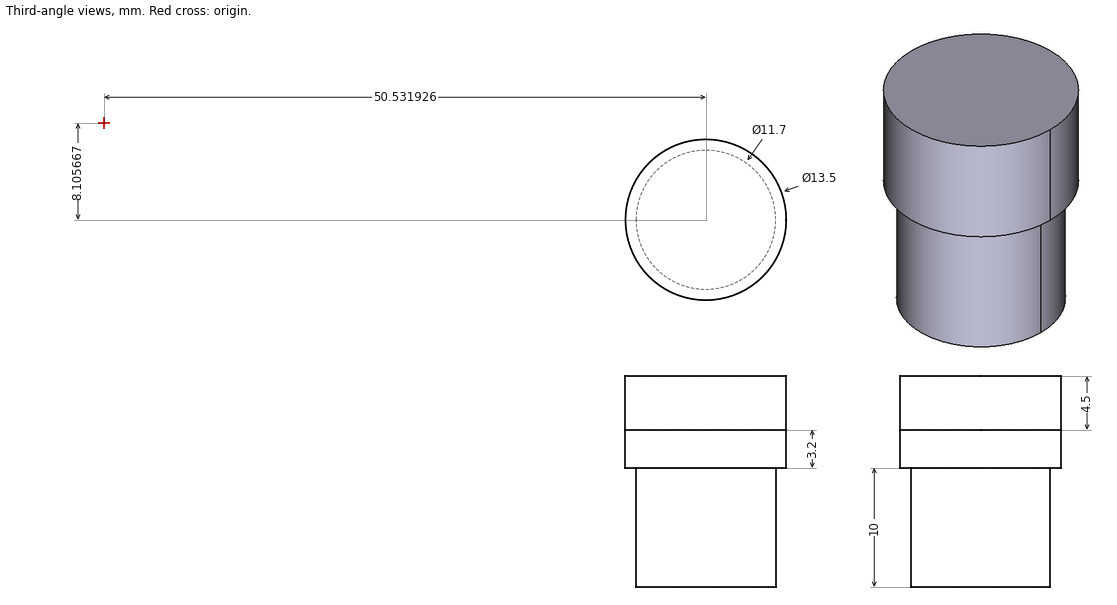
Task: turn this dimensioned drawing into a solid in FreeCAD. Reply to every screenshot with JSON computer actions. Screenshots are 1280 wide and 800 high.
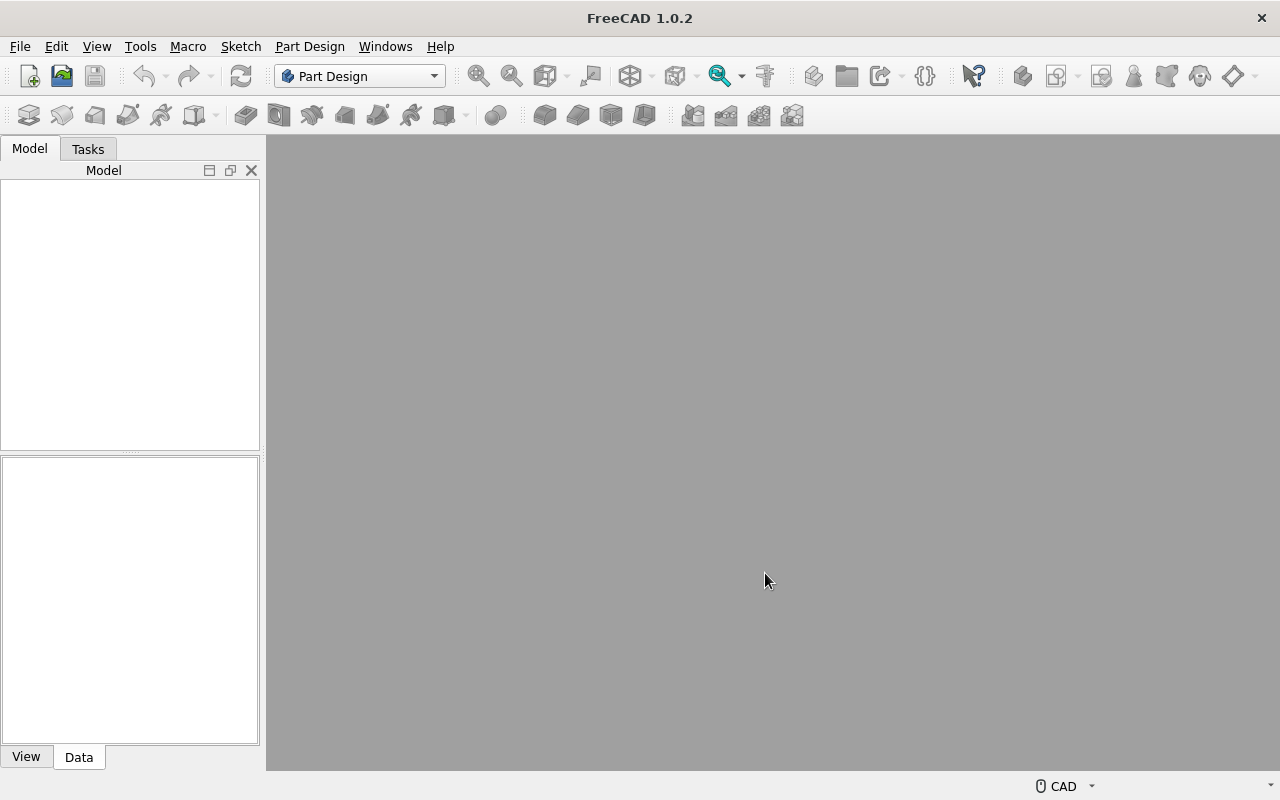
{"action": "key", "text": "ctrl+n"}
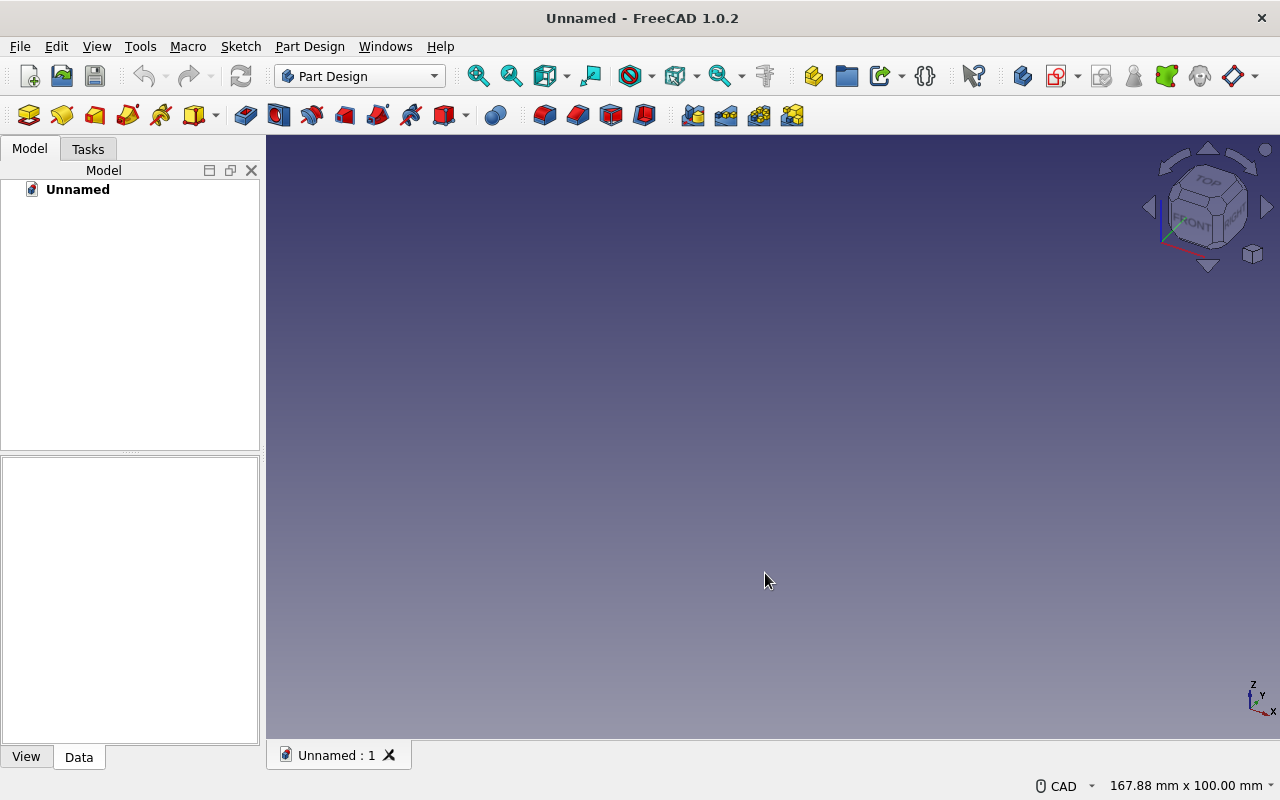
{"action": "left_click", "coordinate": [1056, 76]}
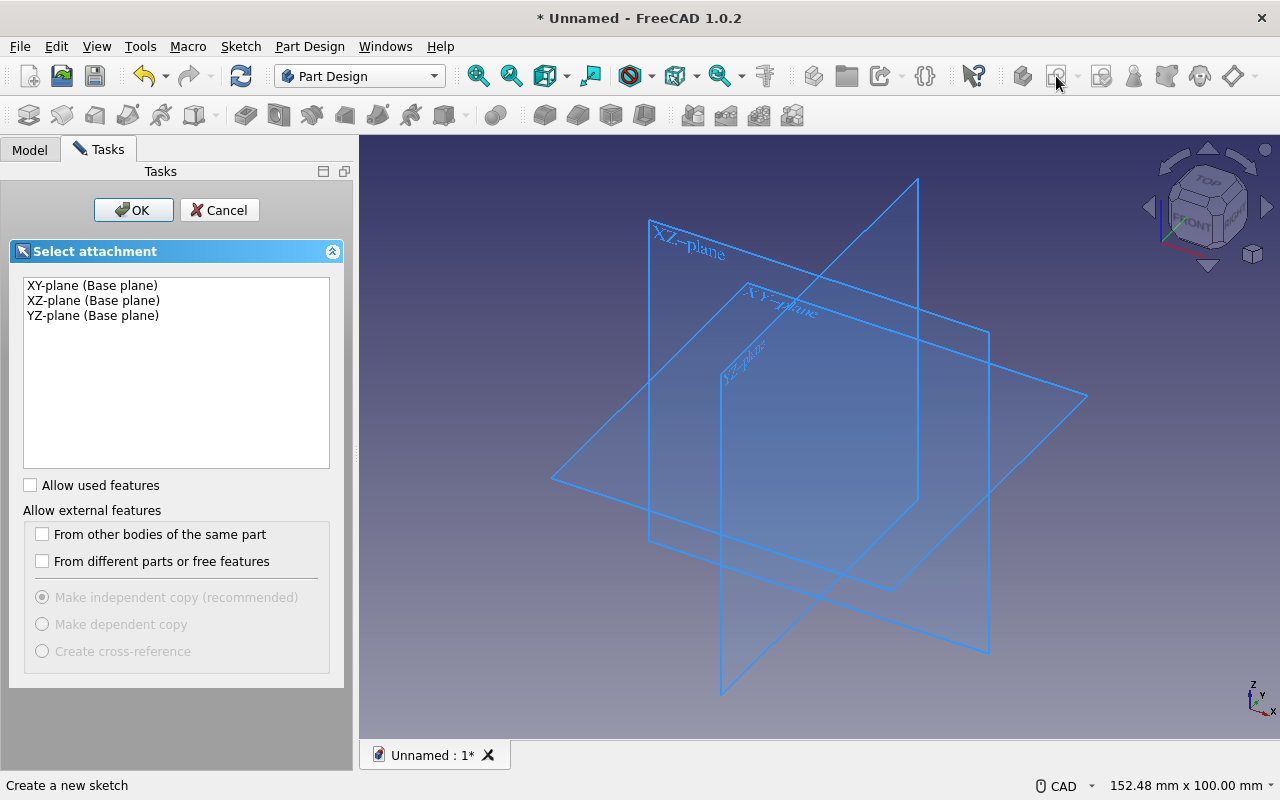
{"action": "left_click", "coordinate": [84, 286]}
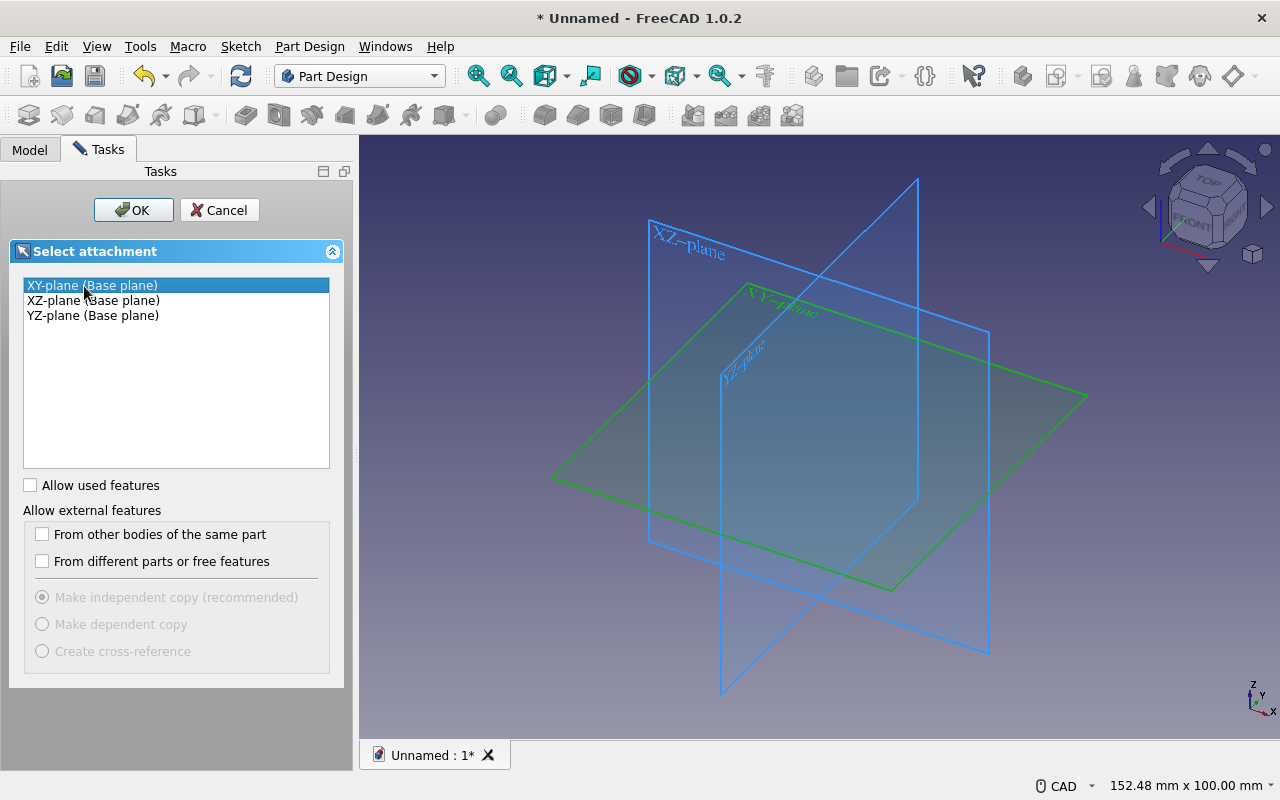
{"action": "left_click", "coordinate": [134, 210]}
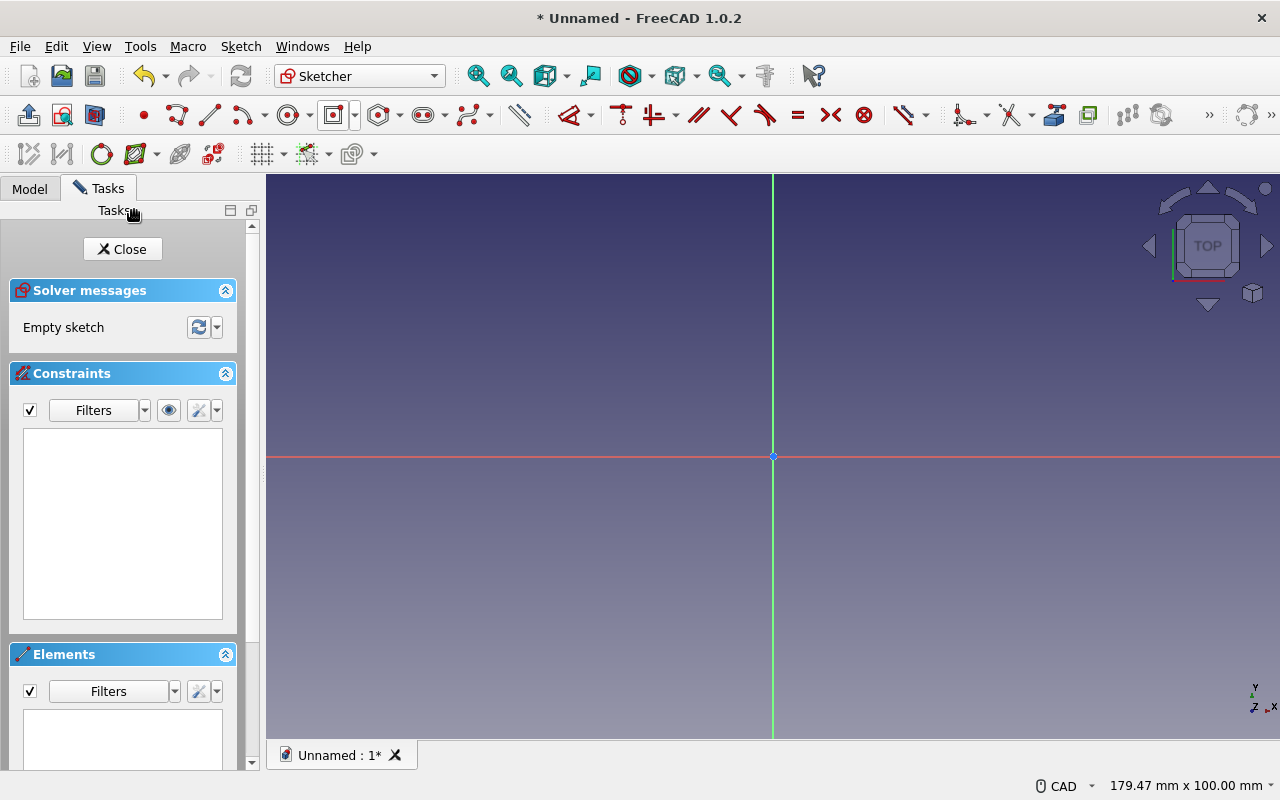
{"action": "scroll", "coordinate": [1115, 514], "scroll_direction": "up", "scroll_amount": 8}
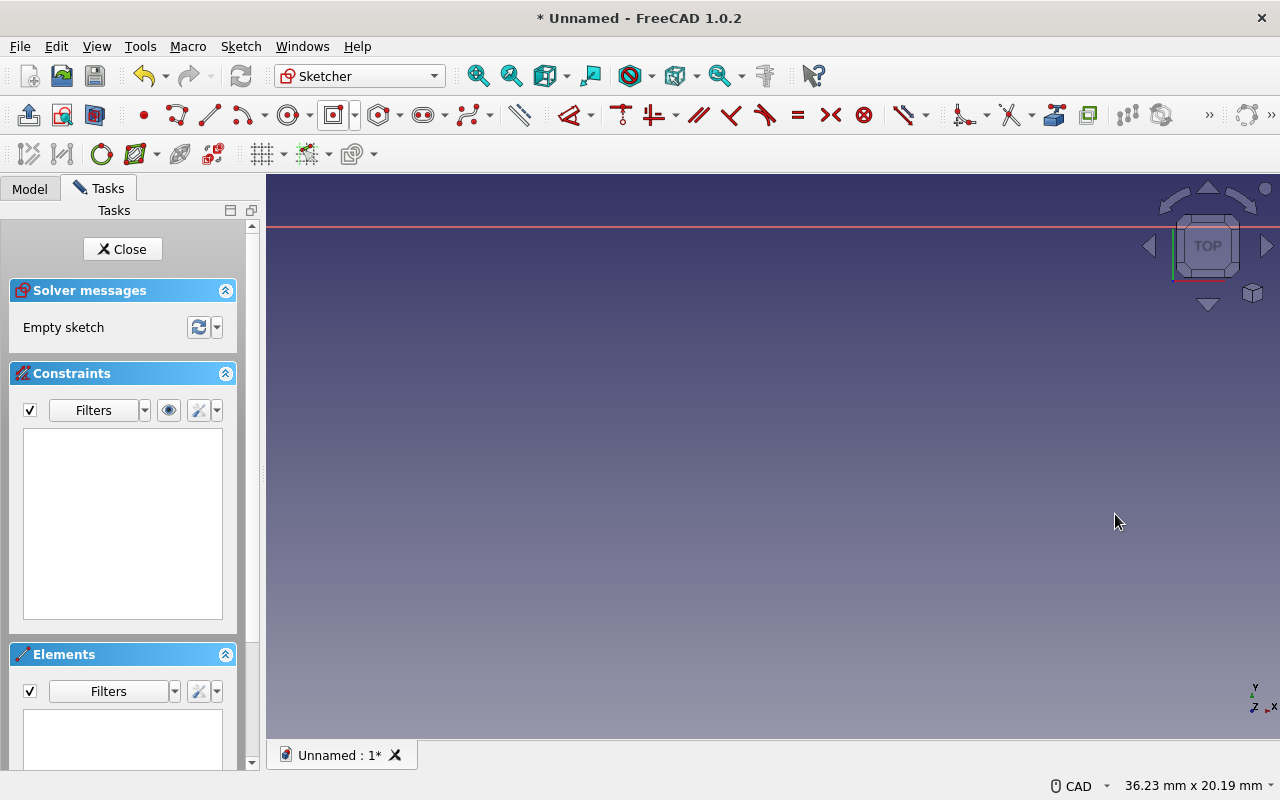
{"action": "left_click", "coordinate": [288, 116]}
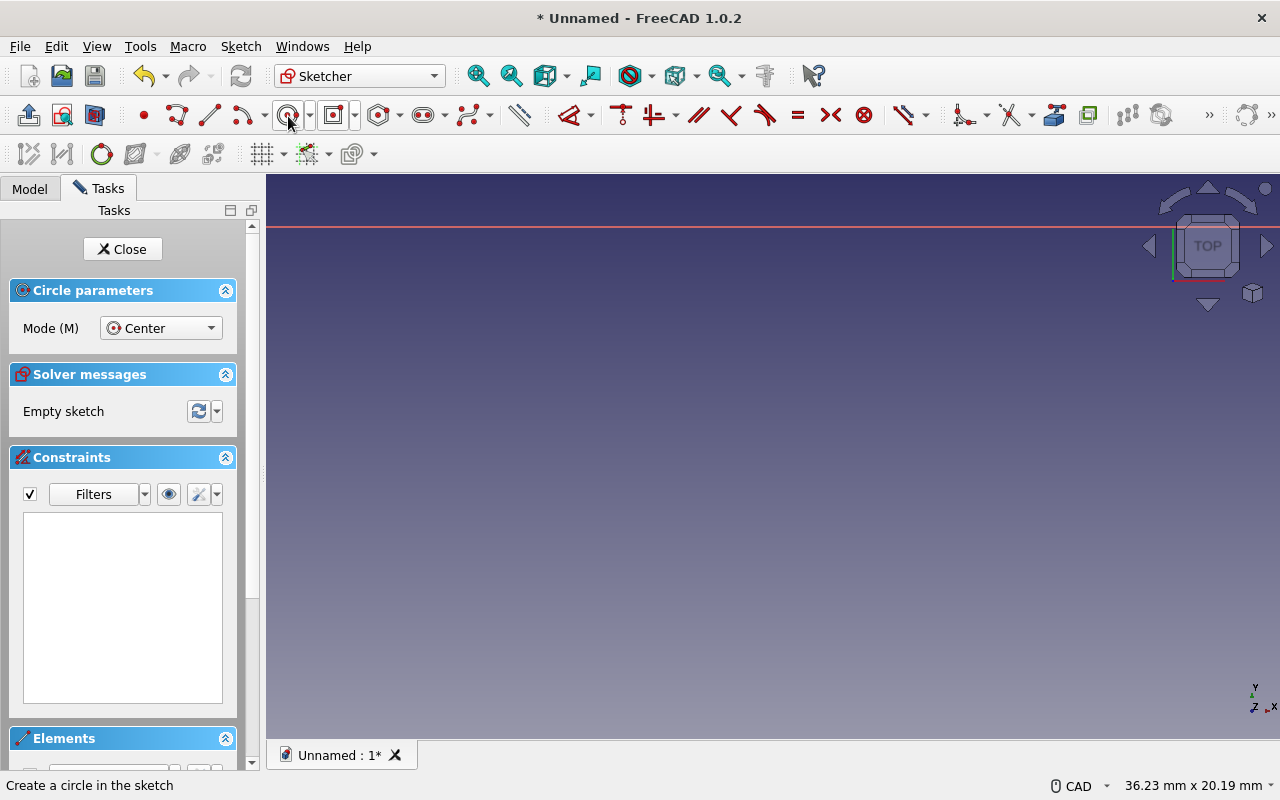
{"action": "left_click", "coordinate": [832, 454]}
{"action": "mouse_move", "coordinate": [965, 320]}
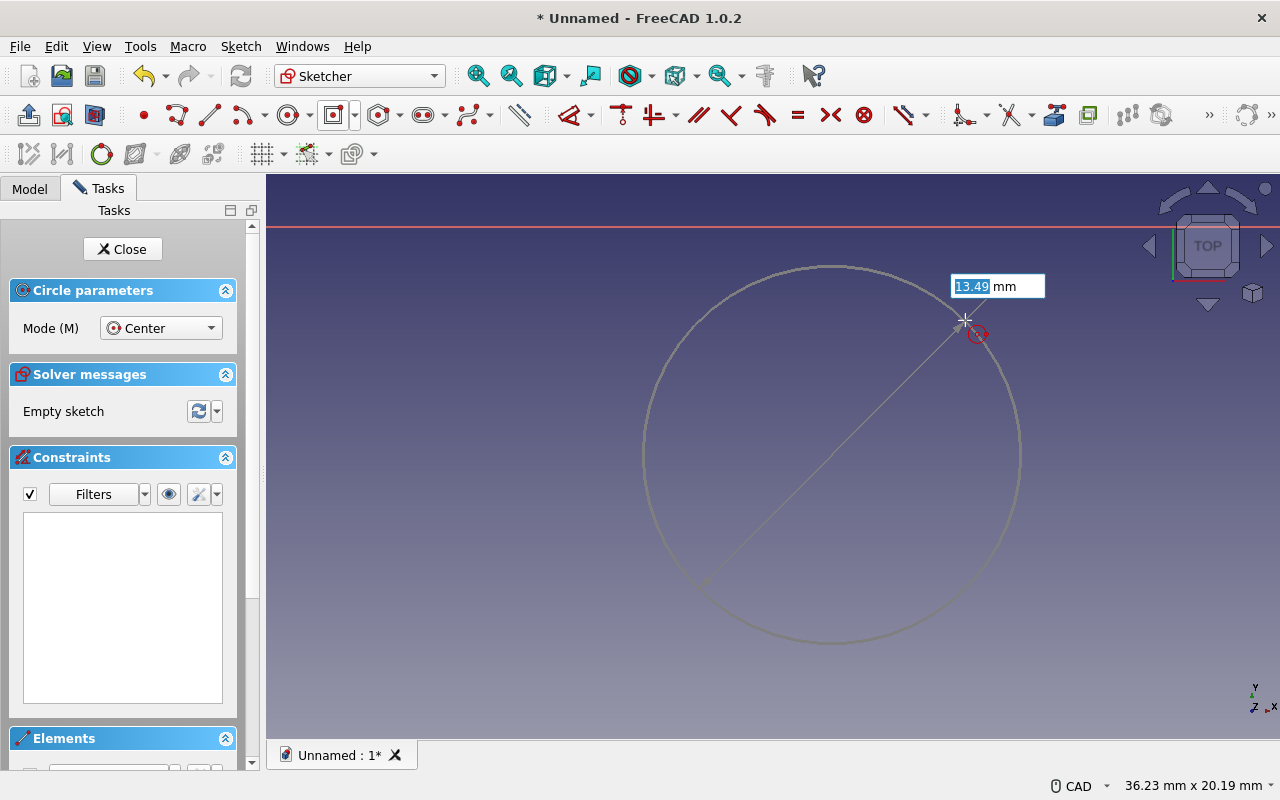
{"action": "type", "text": "13.5"}
{"action": "key", "text": "Return"}
{"action": "key", "text": "Escape"}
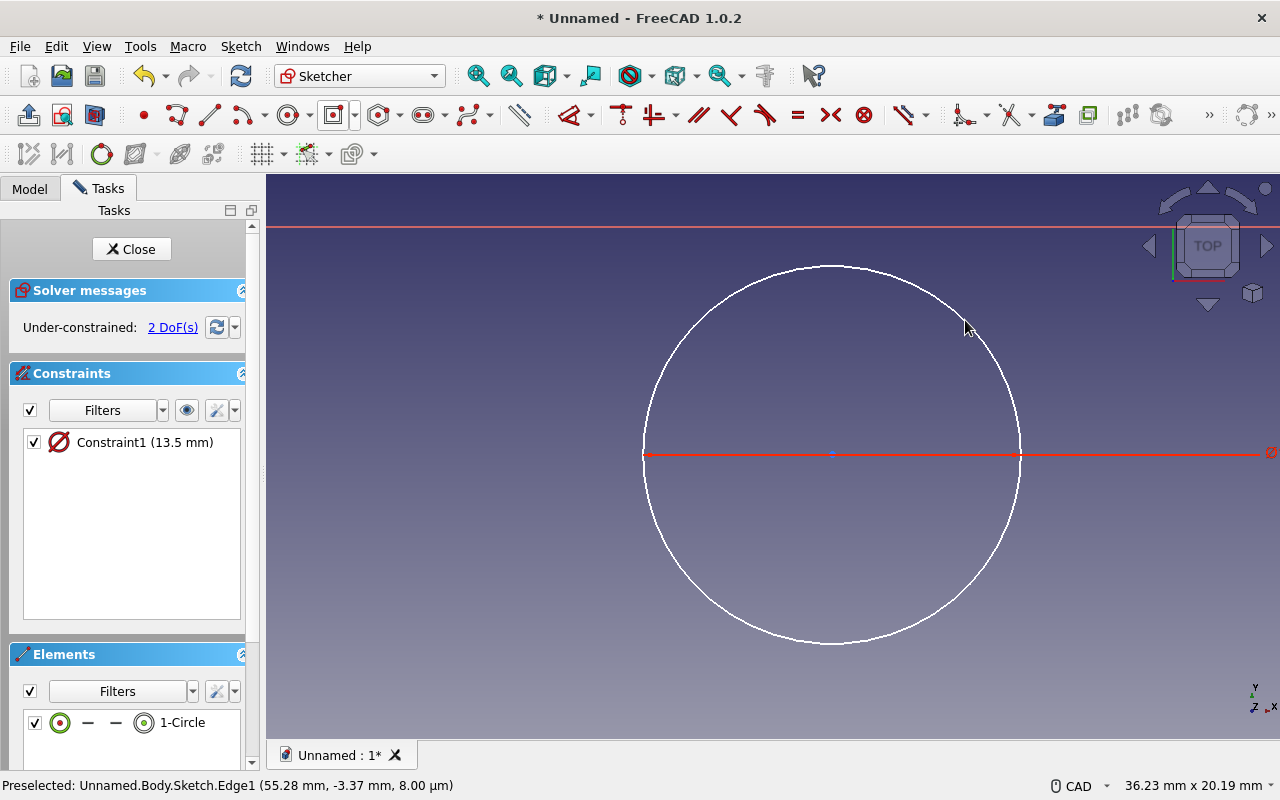
{"action": "key", "text": "d"}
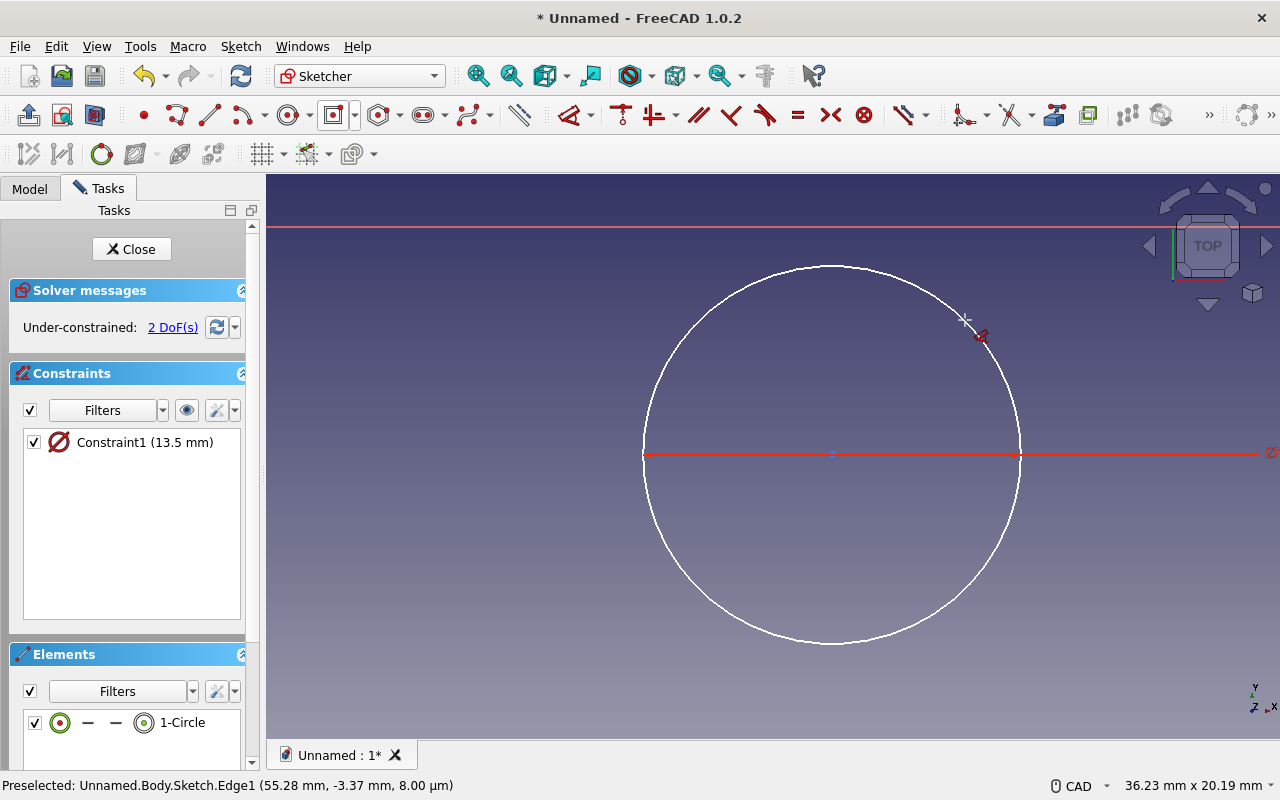
{"action": "left_click", "coordinate": [832, 455]}
{"action": "left_click", "coordinate": [866, 341]}